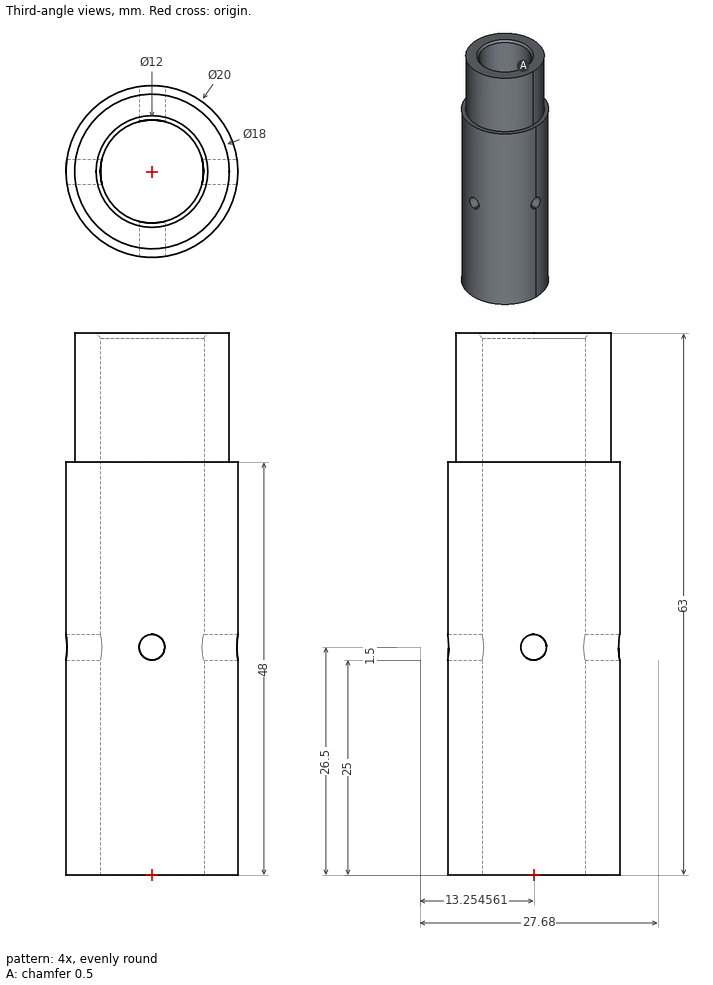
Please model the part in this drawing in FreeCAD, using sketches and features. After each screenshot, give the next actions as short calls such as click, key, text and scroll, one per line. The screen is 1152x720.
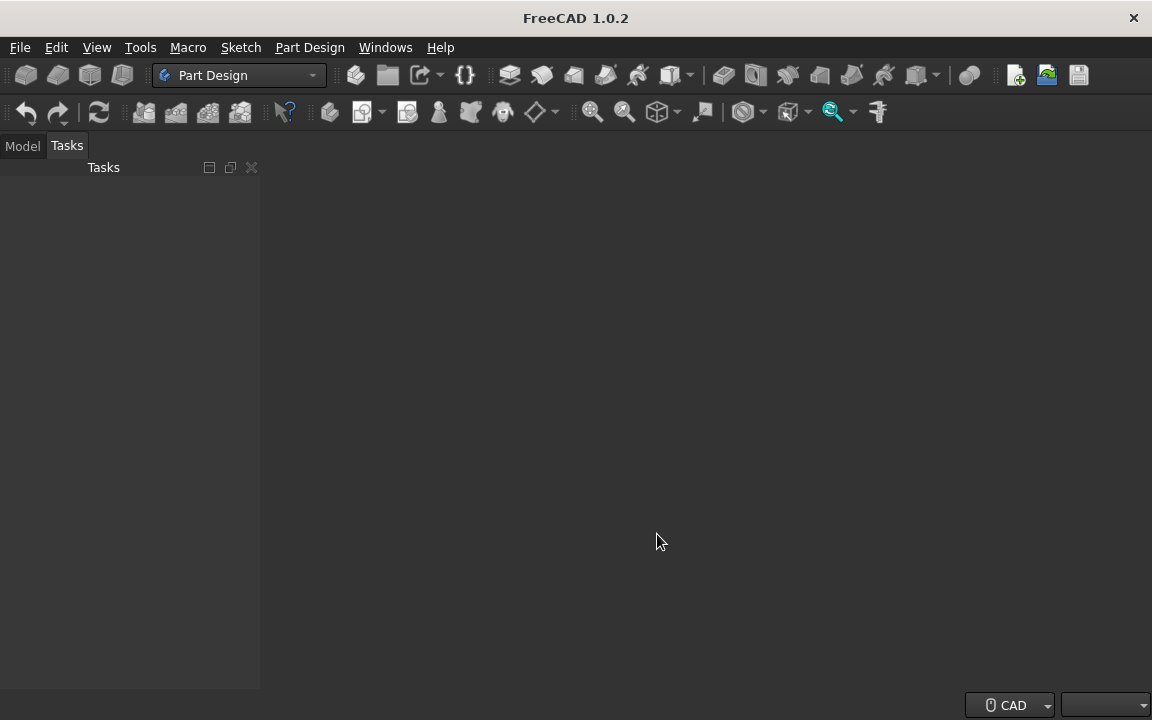
click(1016, 76)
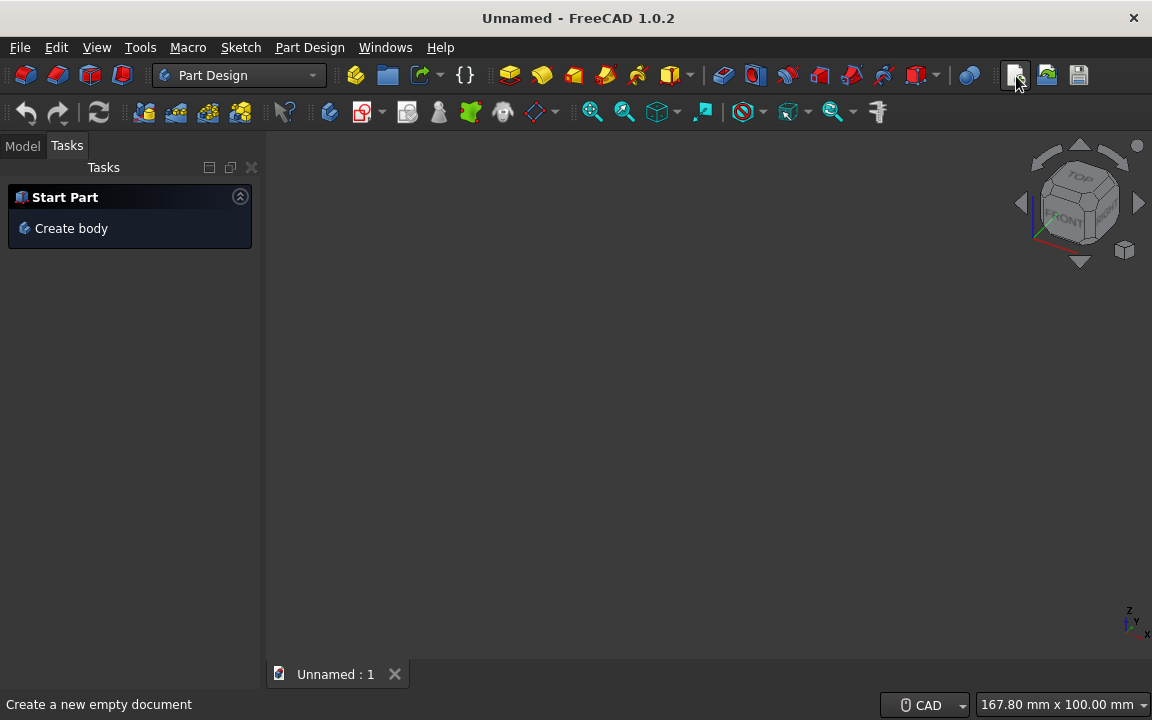
click(362, 112)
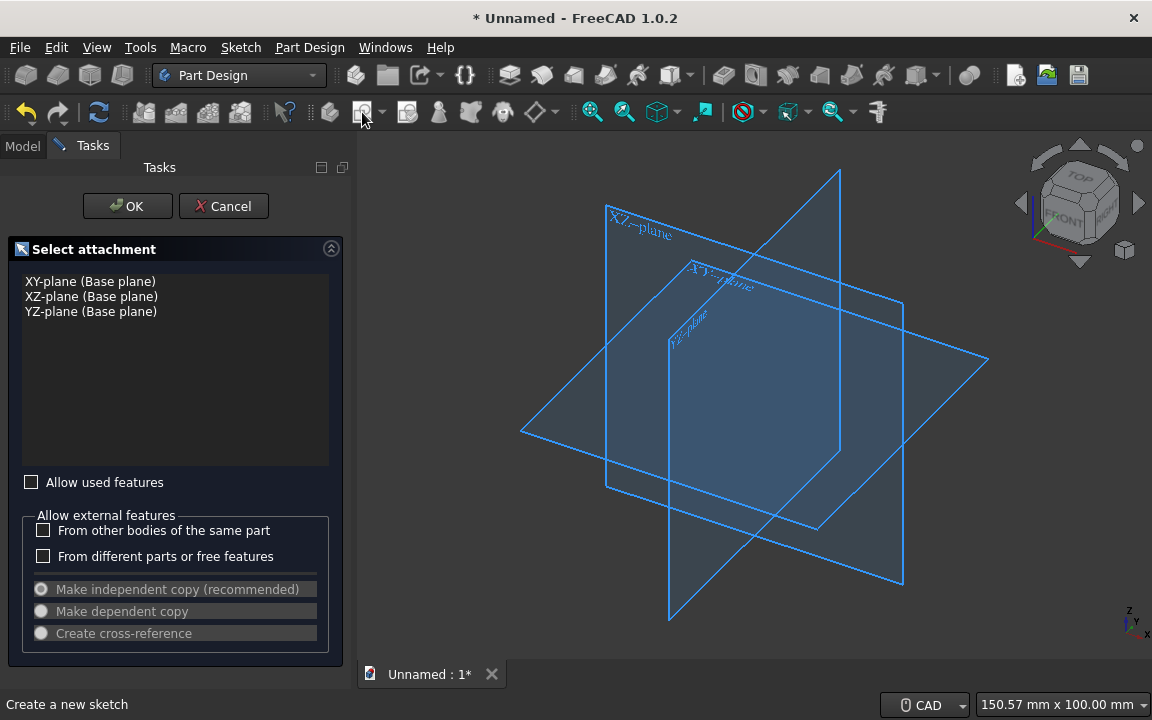
click(82, 282)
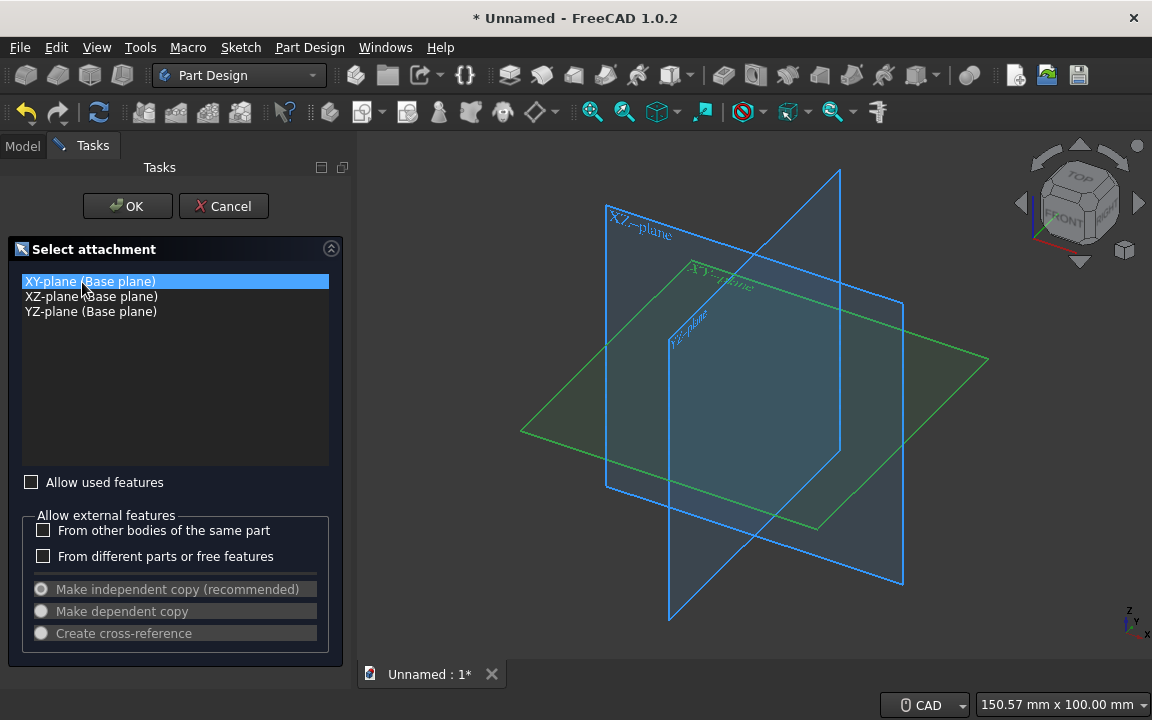
click(128, 206)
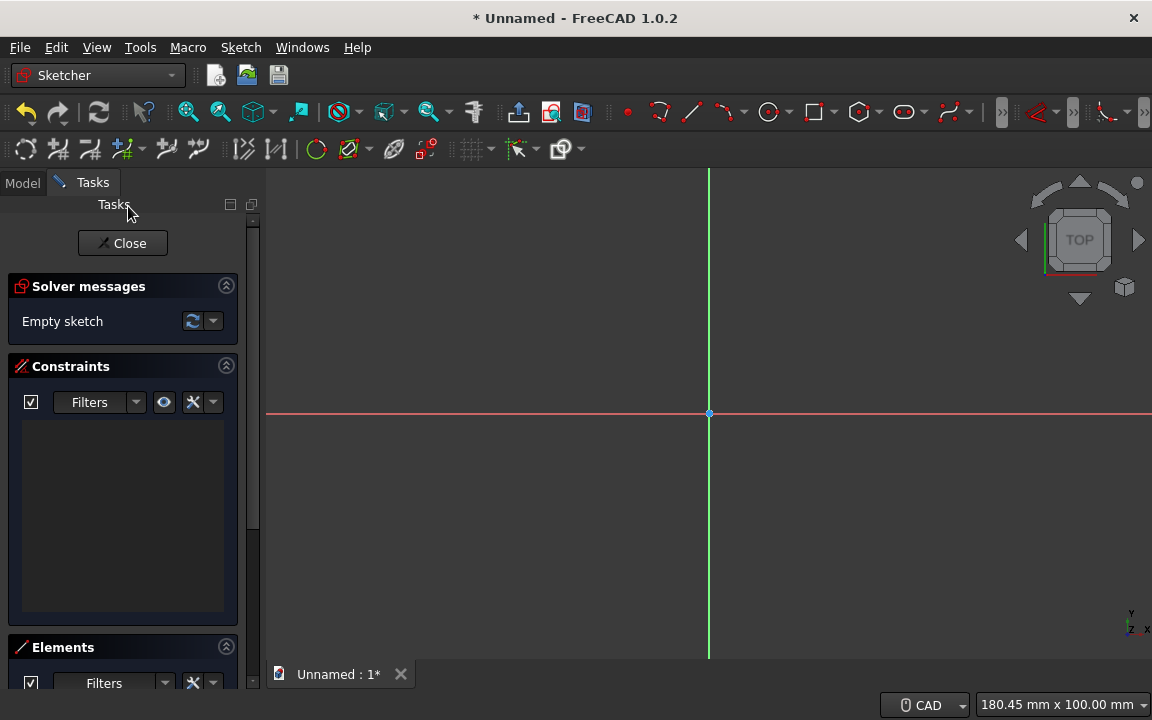
scroll(739, 414, up, 6)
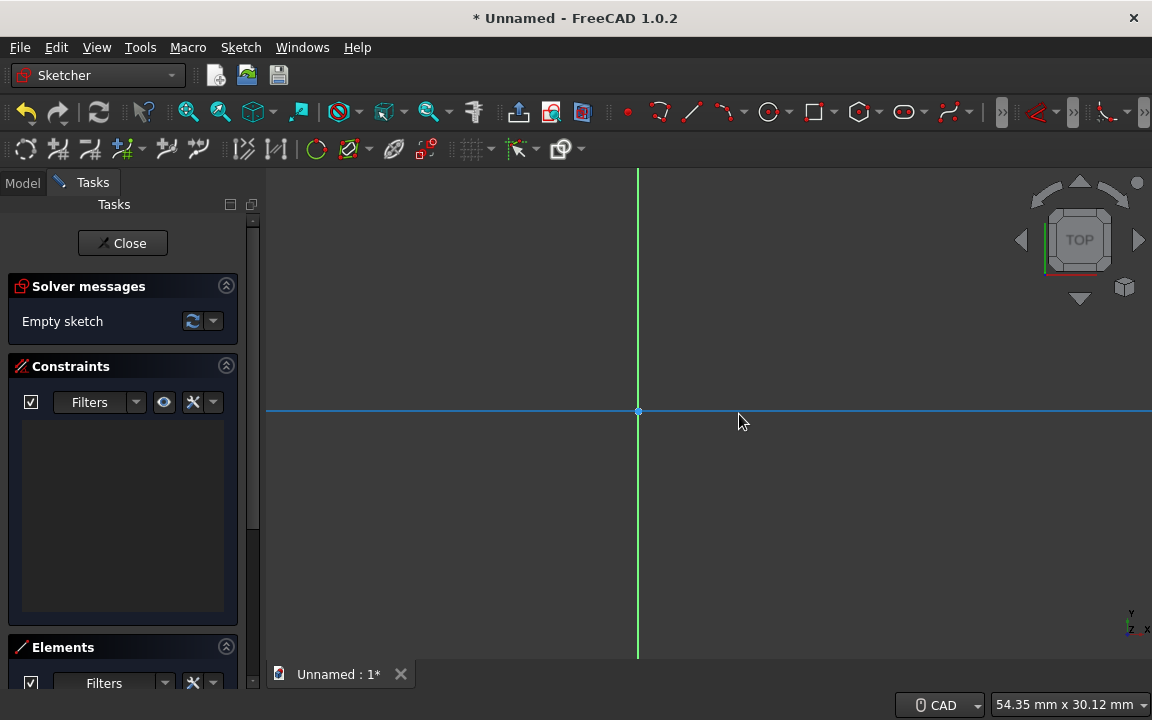
click(770, 112)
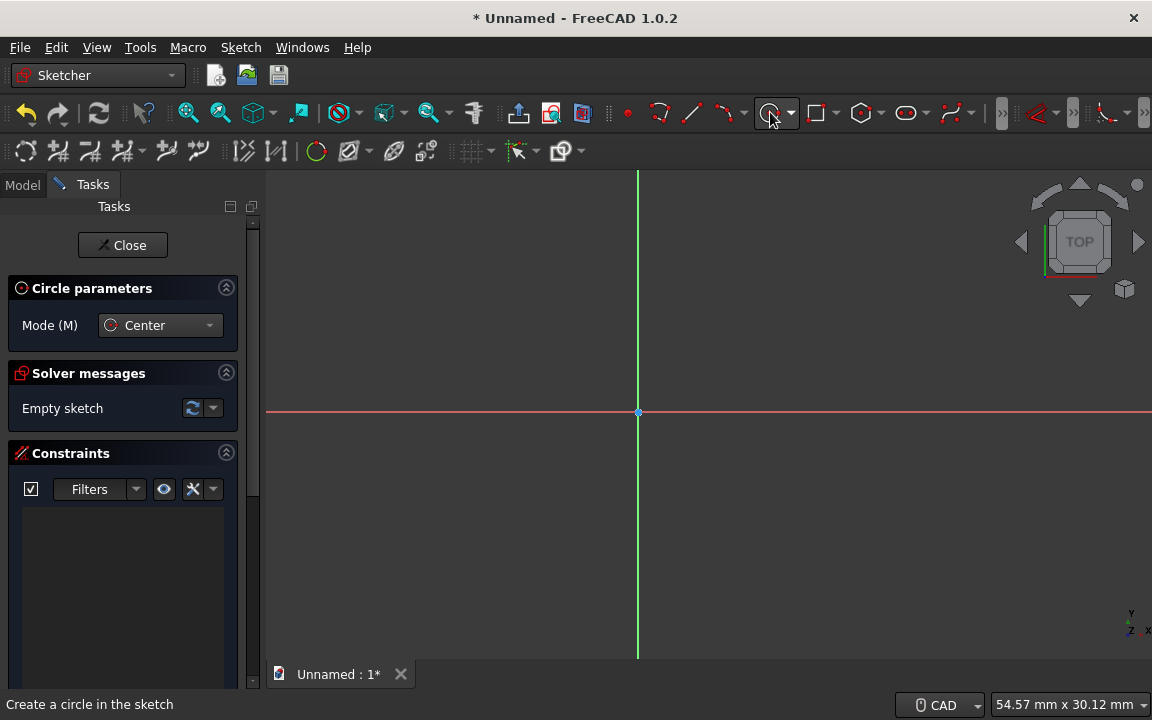
click(638, 412)
click(742, 309)
key(Escape)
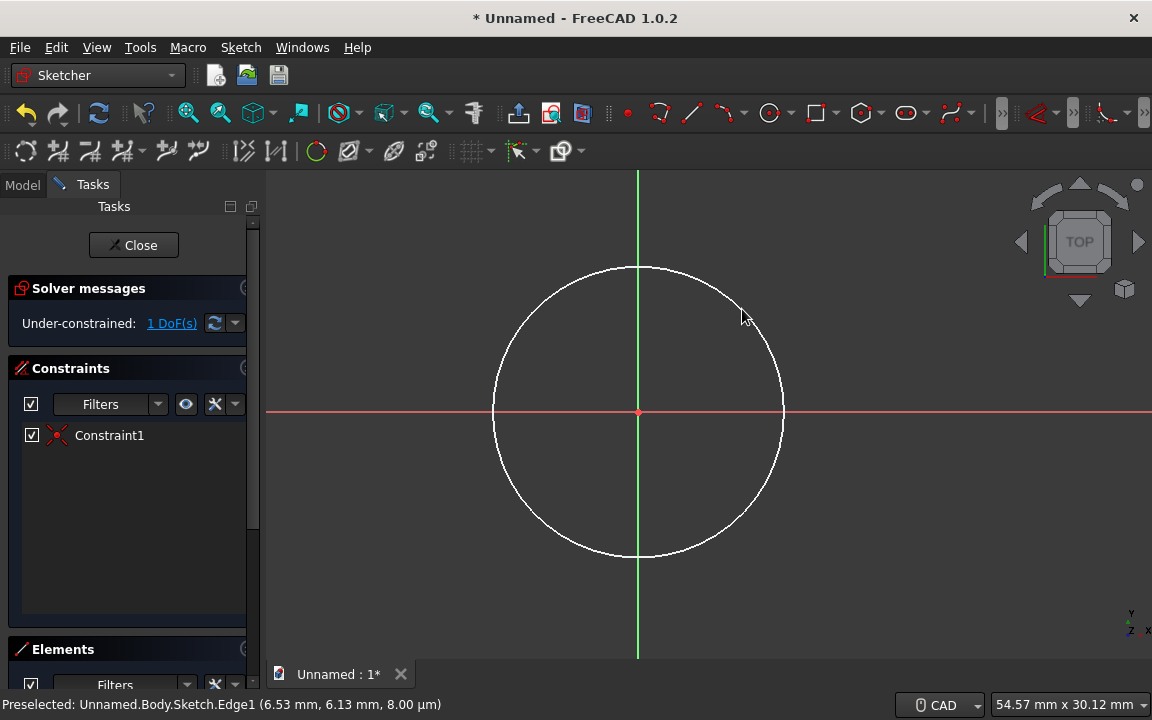
click(1036, 114)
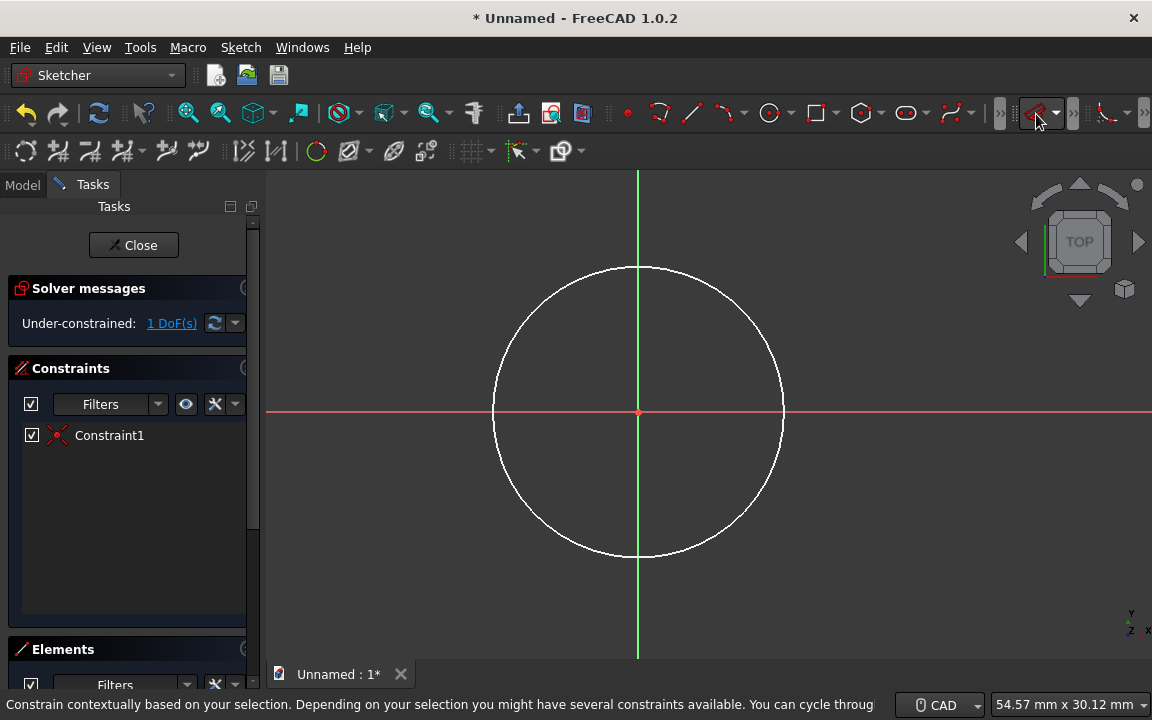
click(741, 309)
click(764, 286)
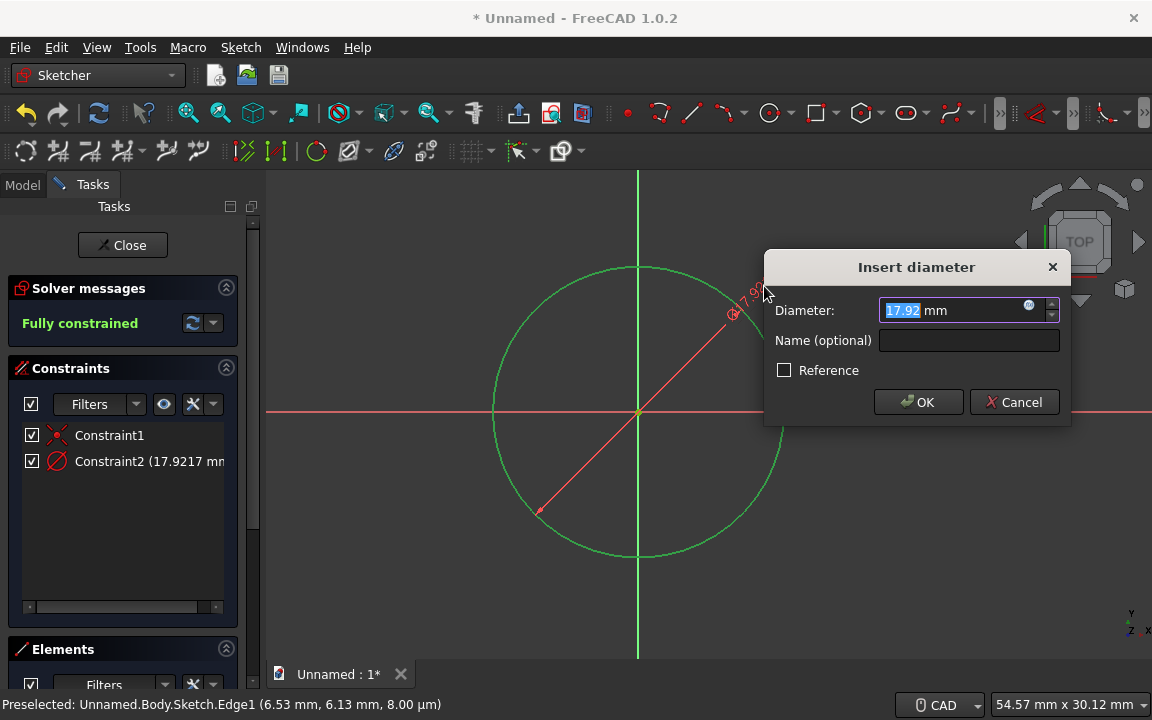
text(18)
key(Return)
key(Escape)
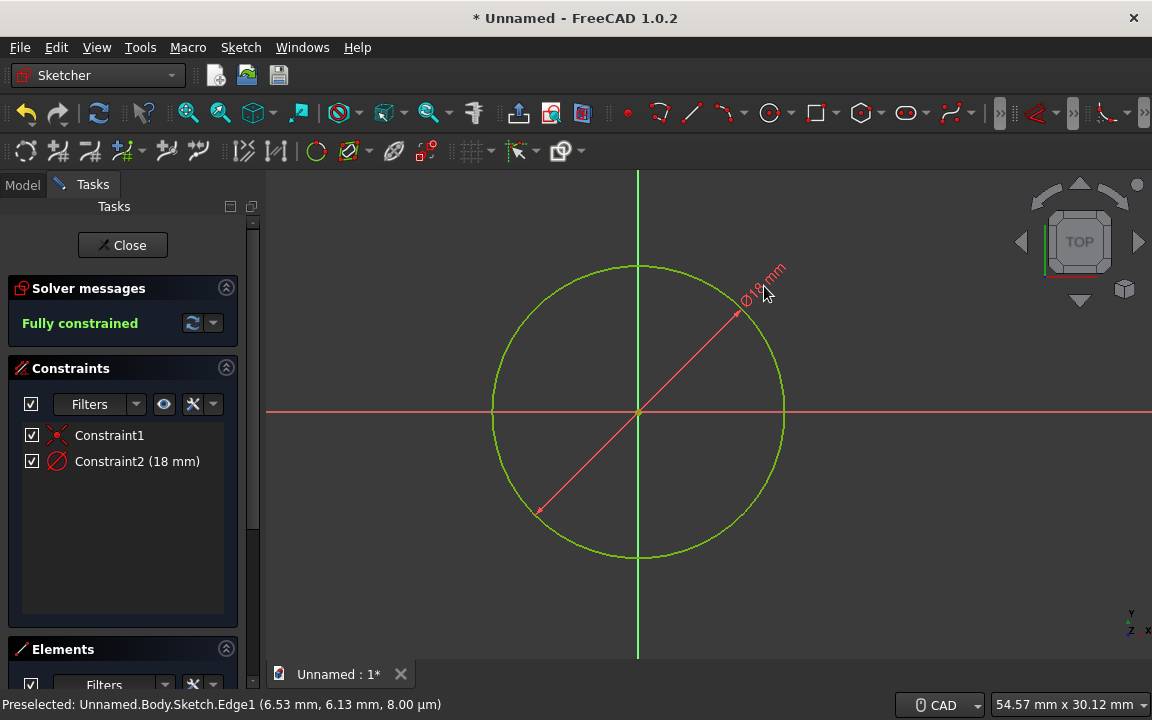
click(123, 245)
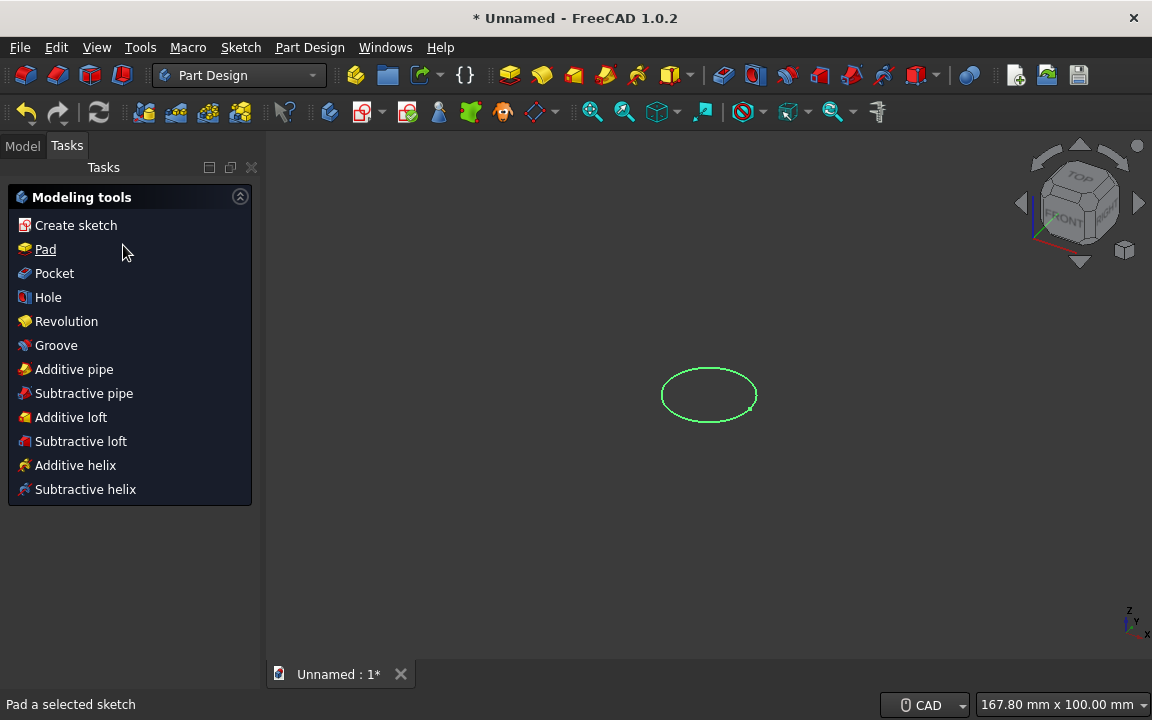
click(510, 76)